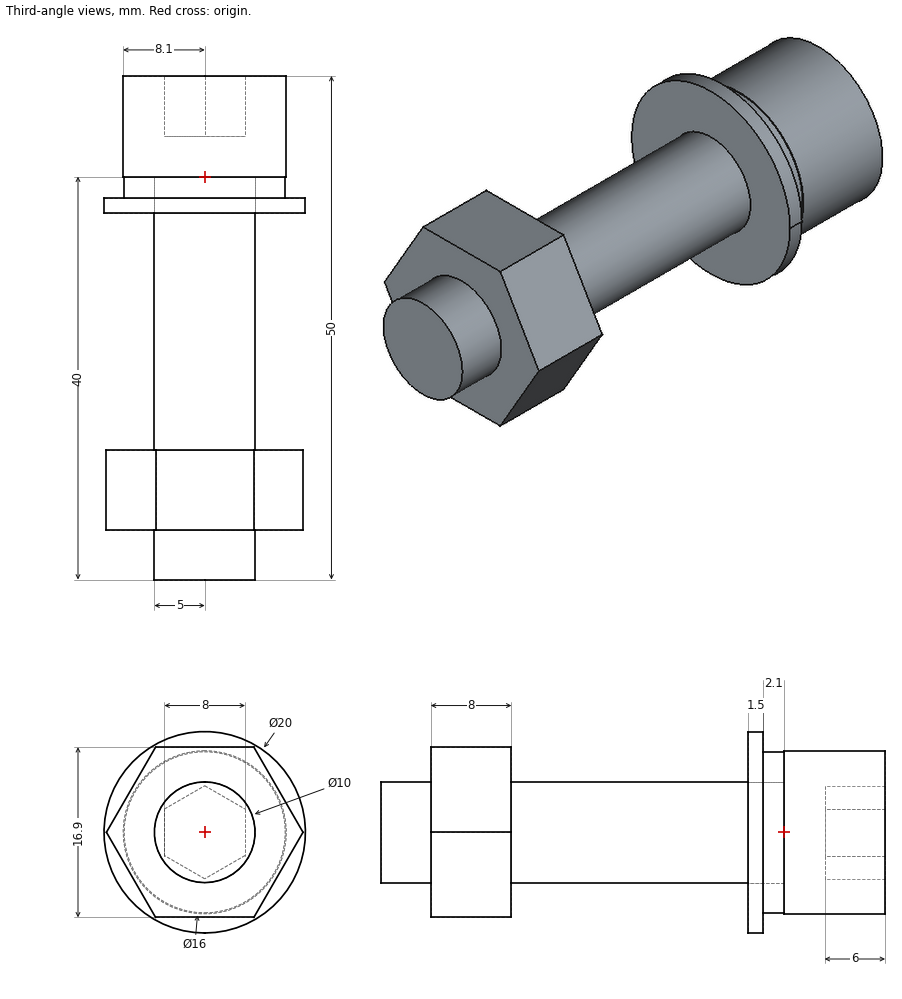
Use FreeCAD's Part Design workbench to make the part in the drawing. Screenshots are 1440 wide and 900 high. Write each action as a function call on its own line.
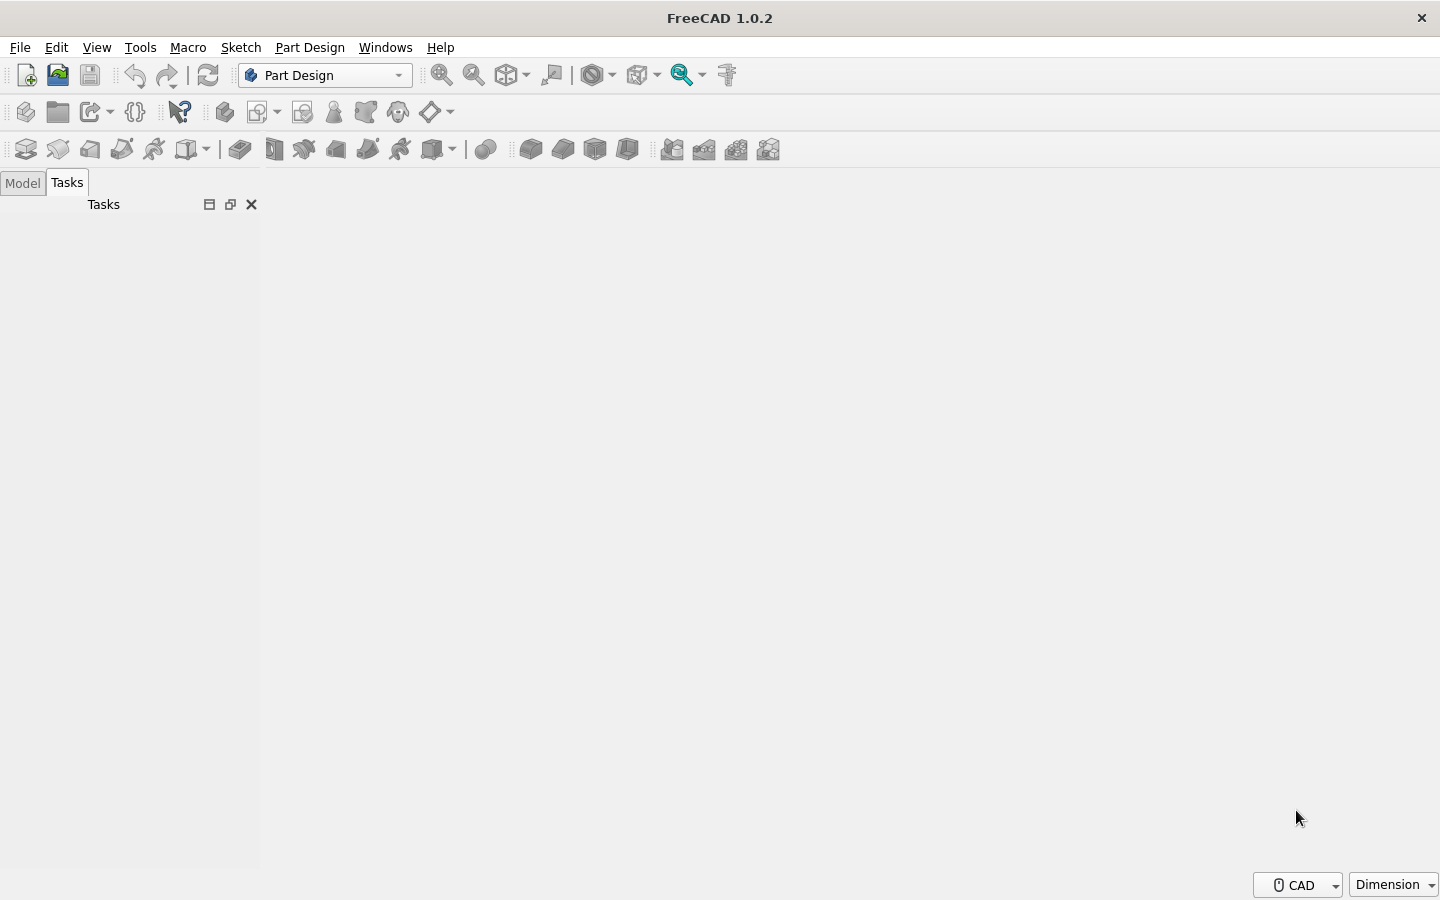
click(26, 76)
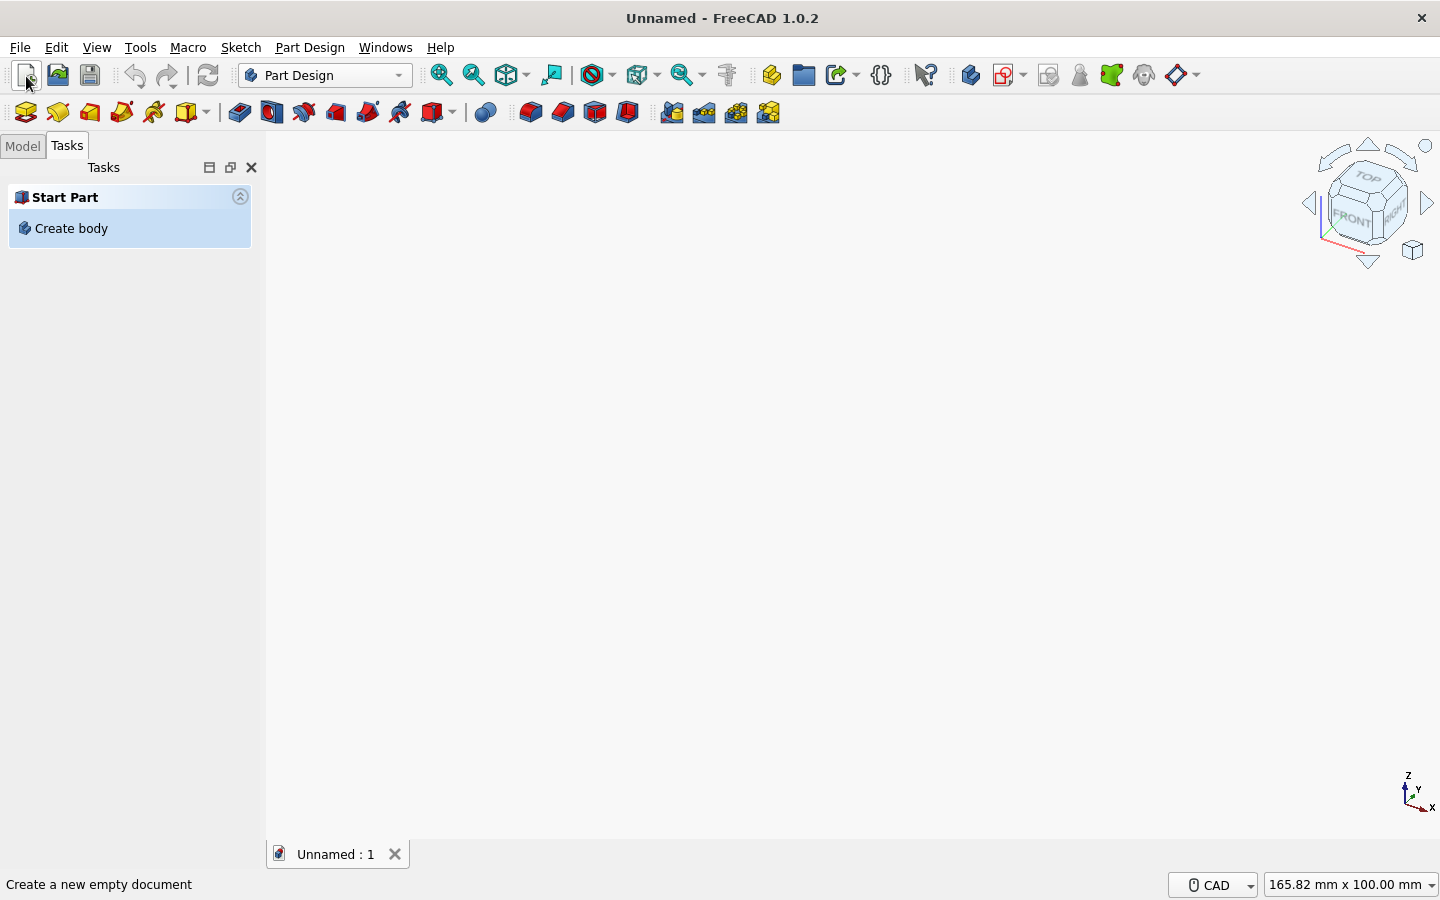
click(1004, 76)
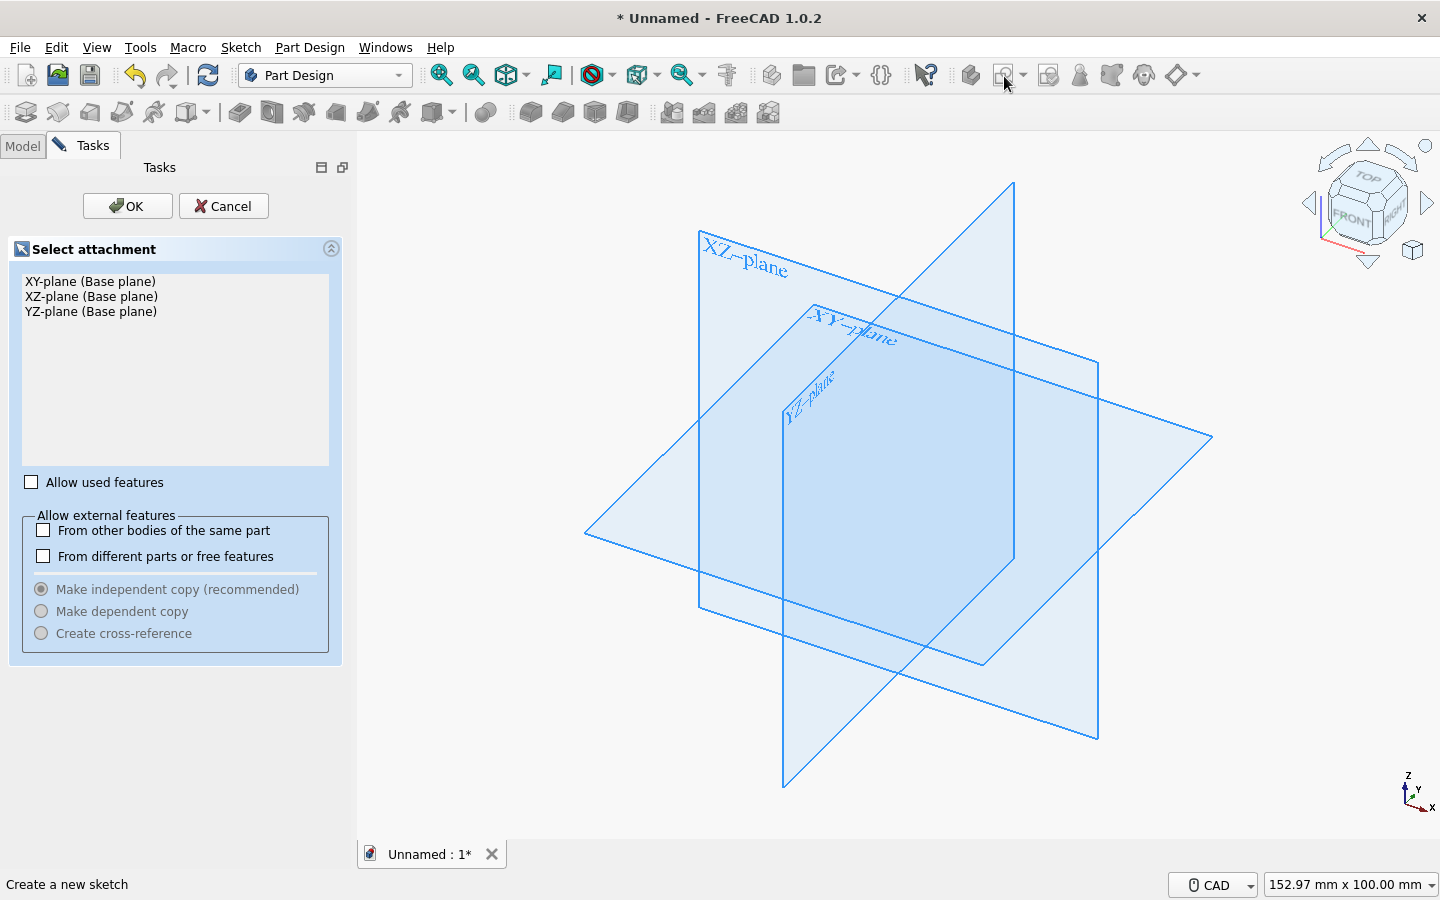
click(82, 282)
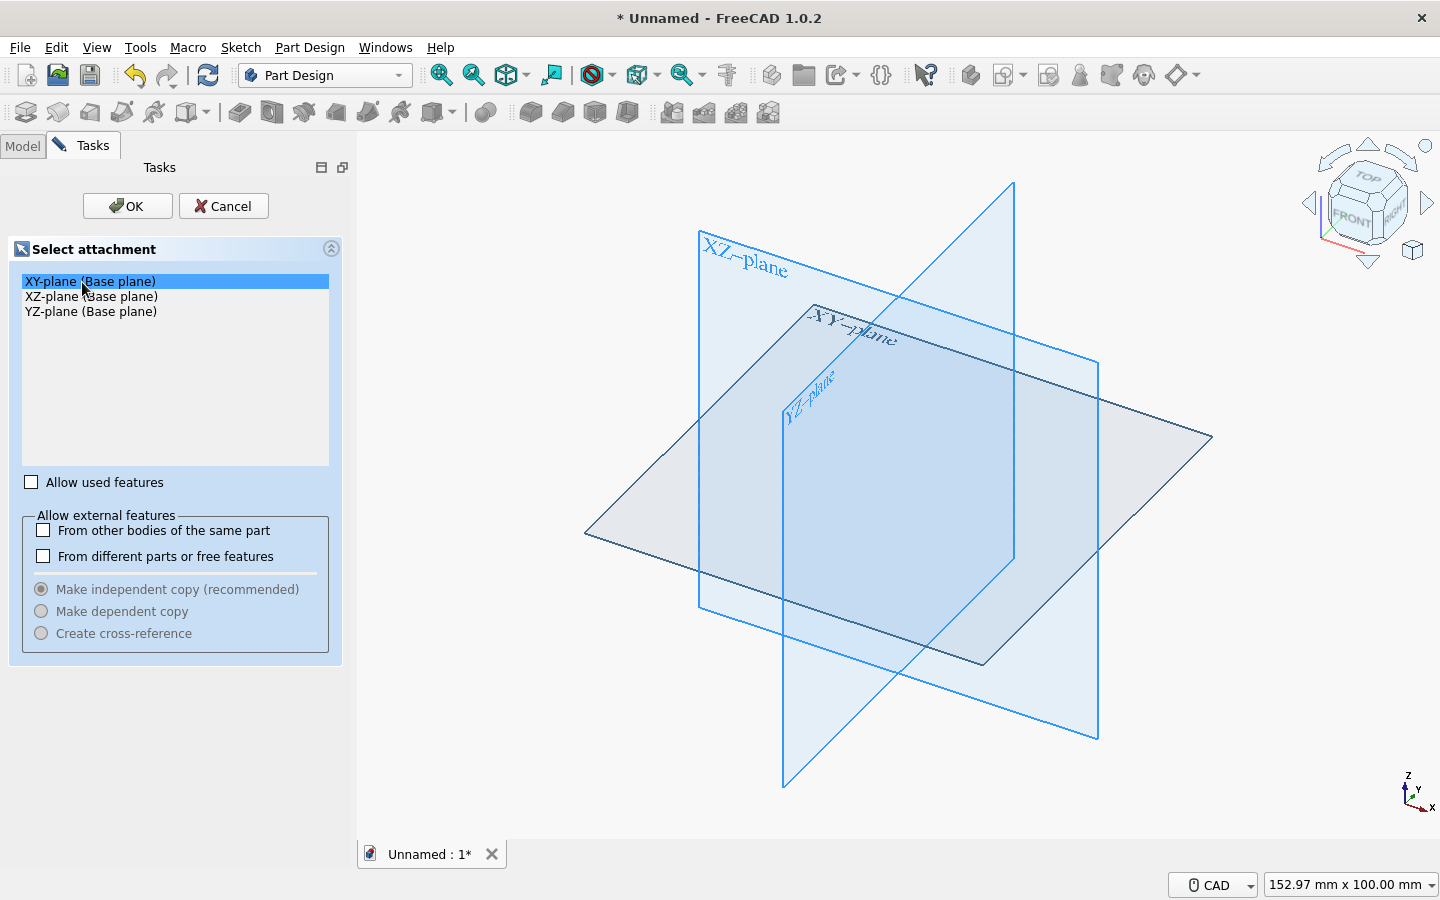
click(128, 206)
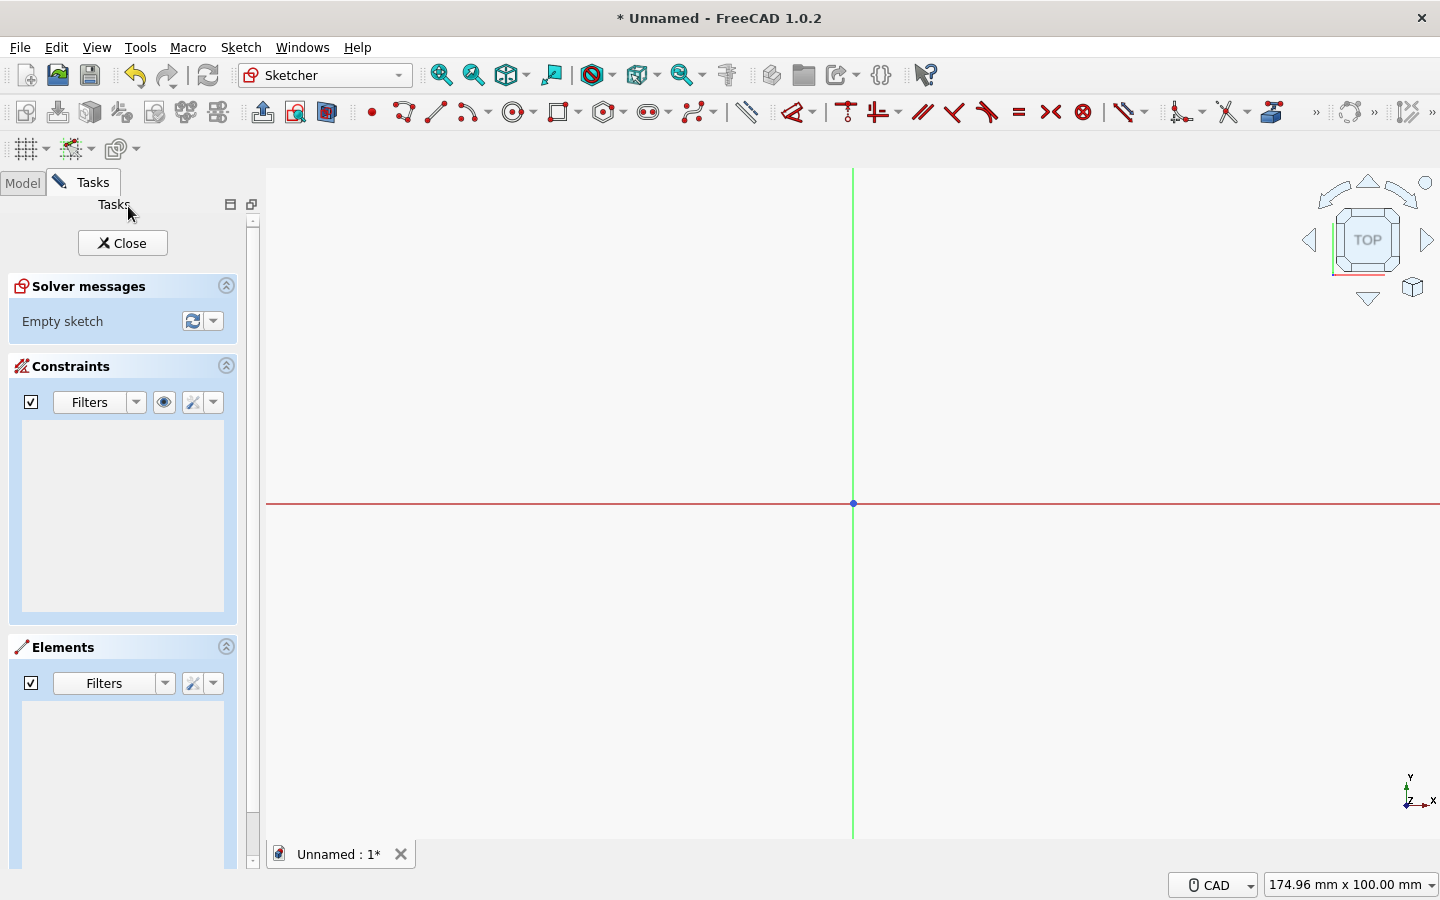
click(404, 112)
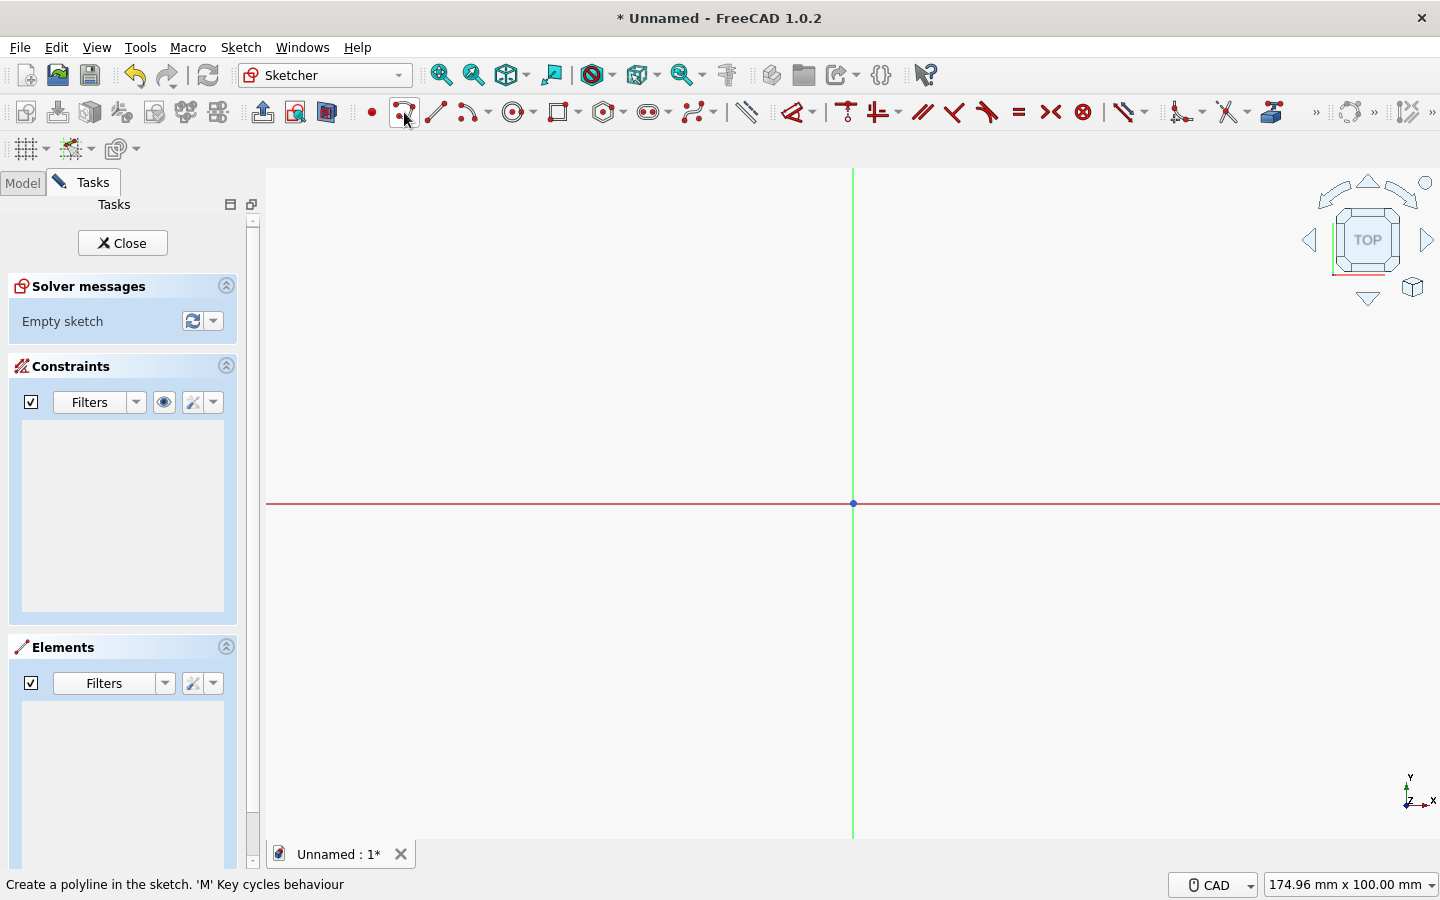
click(819, 504)
click(819, 772)
click(853, 772)
click(844, 436)
click(799, 436)
click(799, 512)
click(819, 504)
key(Escape)
key(Escape)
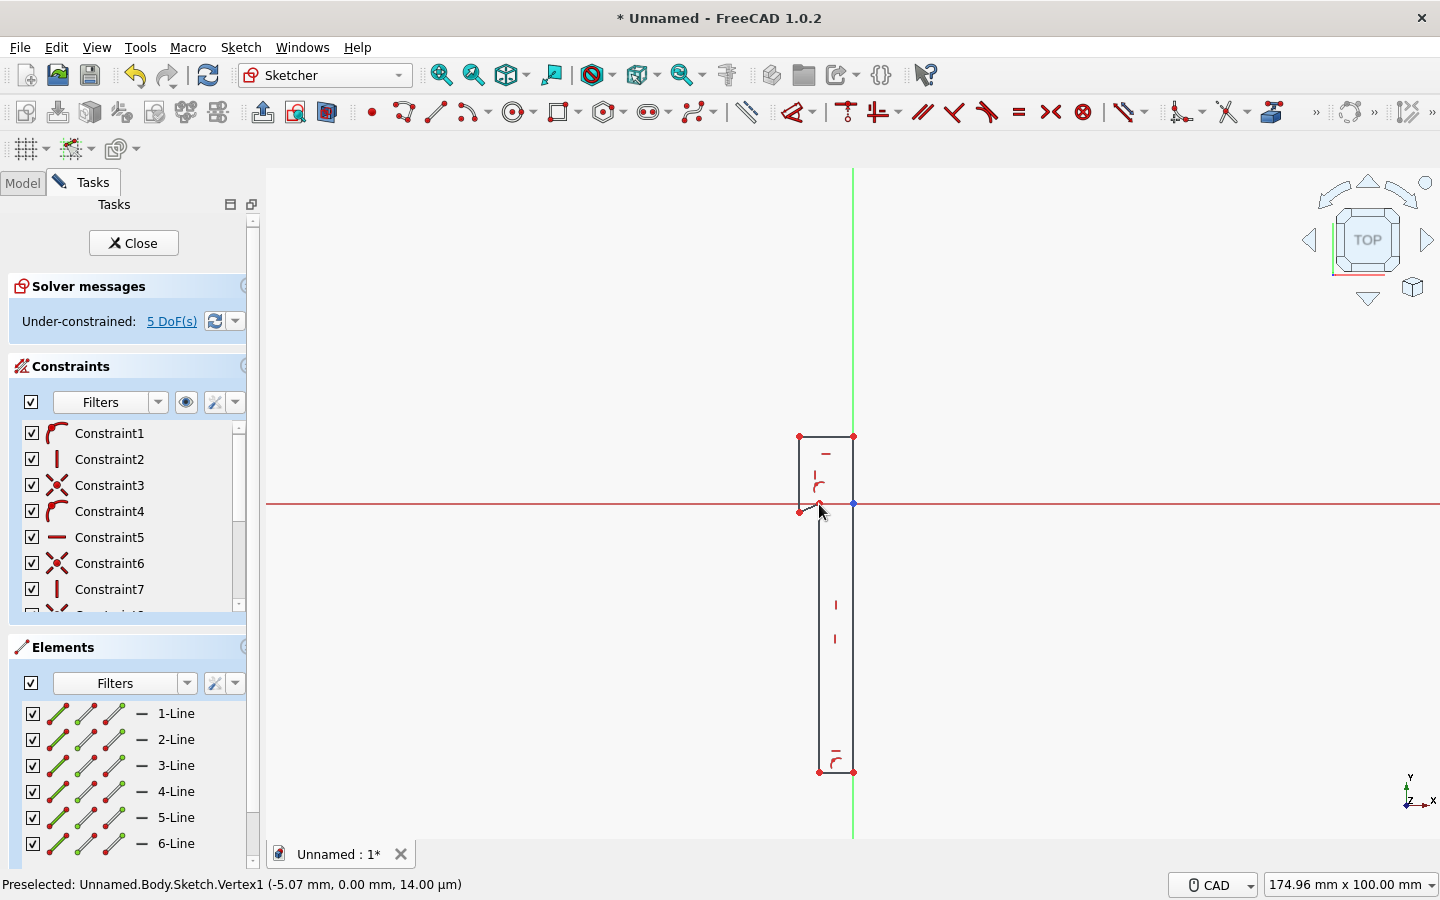
scroll(811, 507, up, 3)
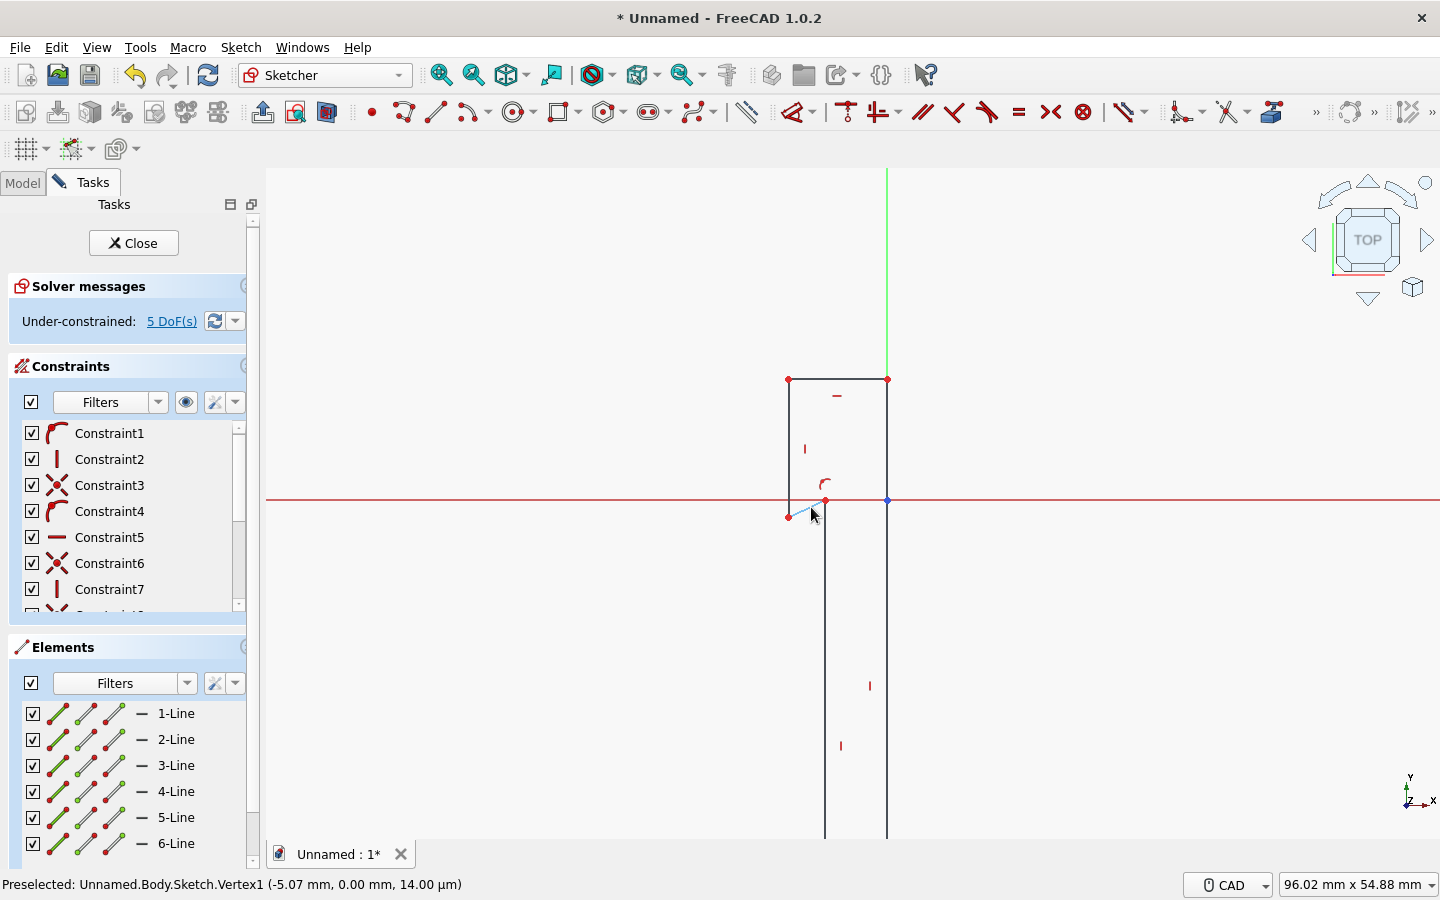
click(811, 507)